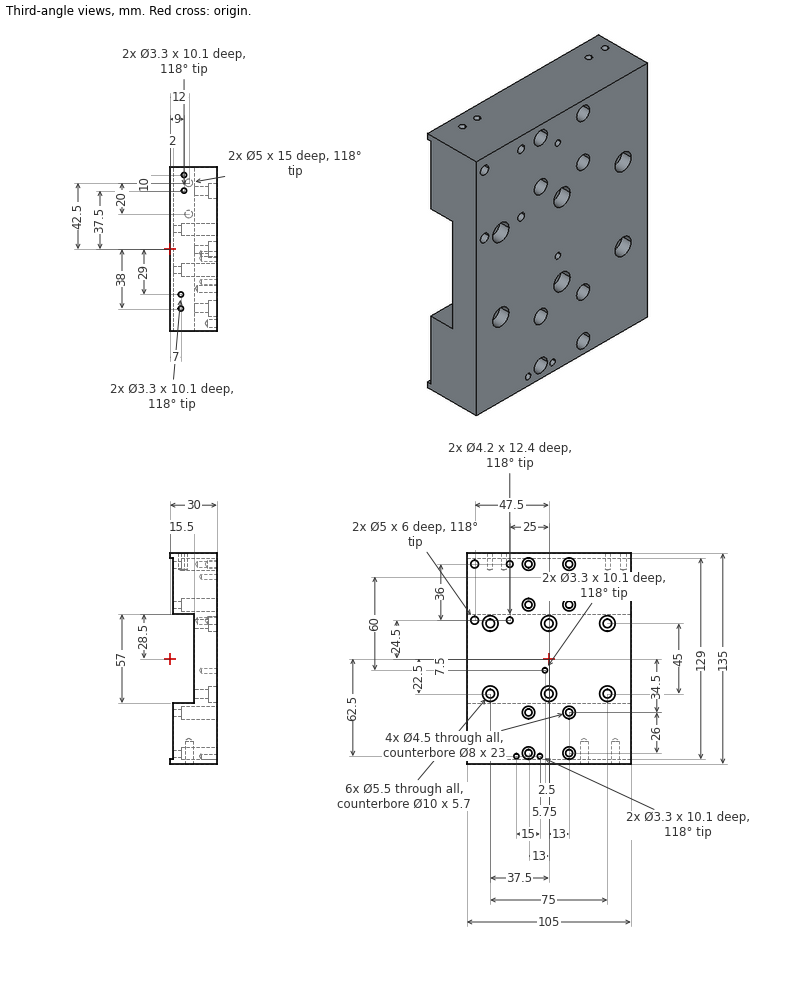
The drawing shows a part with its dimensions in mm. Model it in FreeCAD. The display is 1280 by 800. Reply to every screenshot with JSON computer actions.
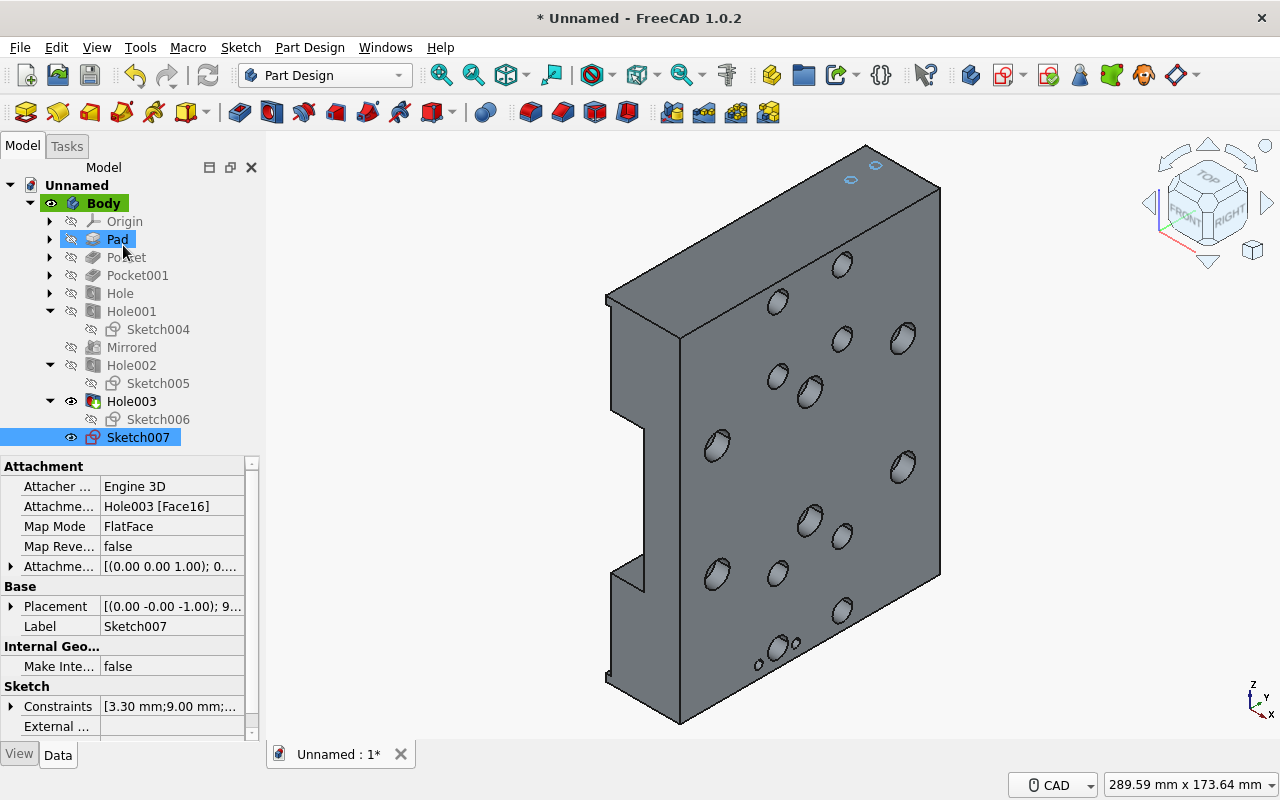
{"action": "left_click", "coordinate": [272, 112]}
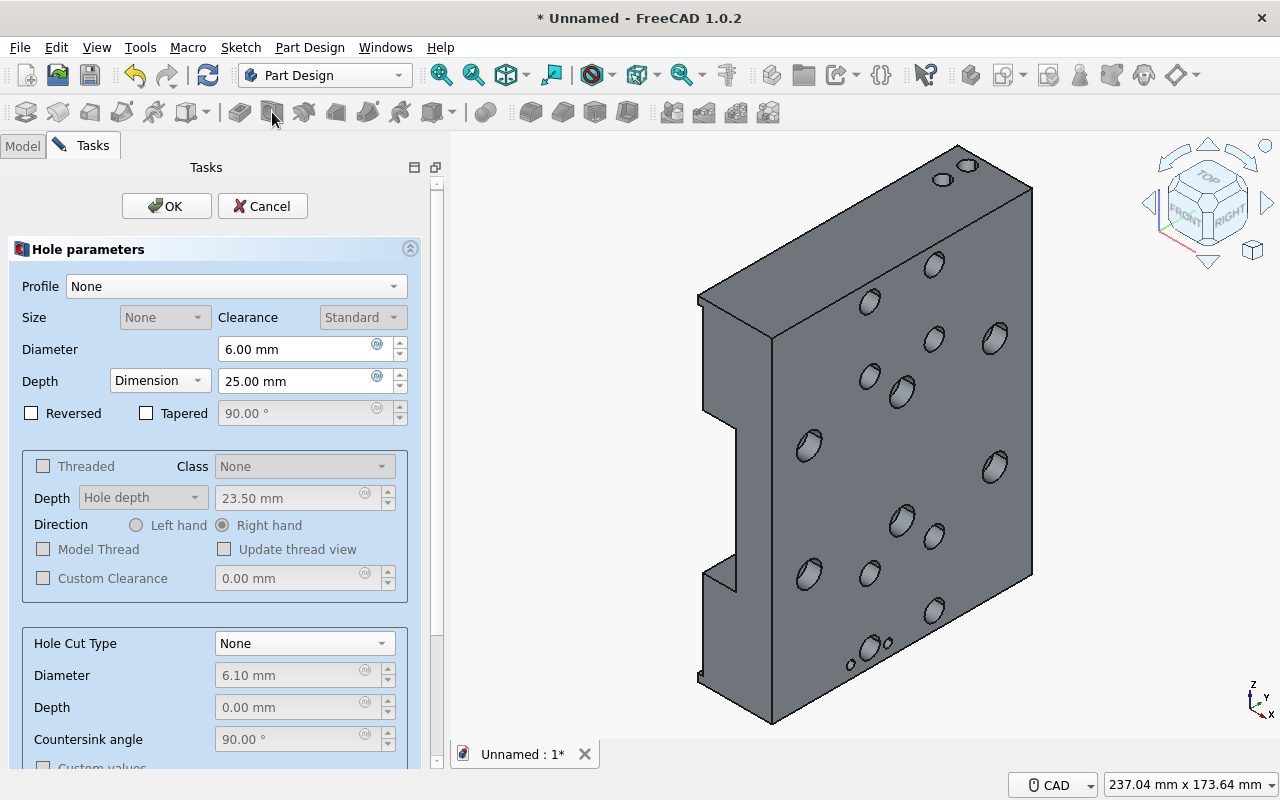
{"action": "triple_click", "coordinate": [305, 349]}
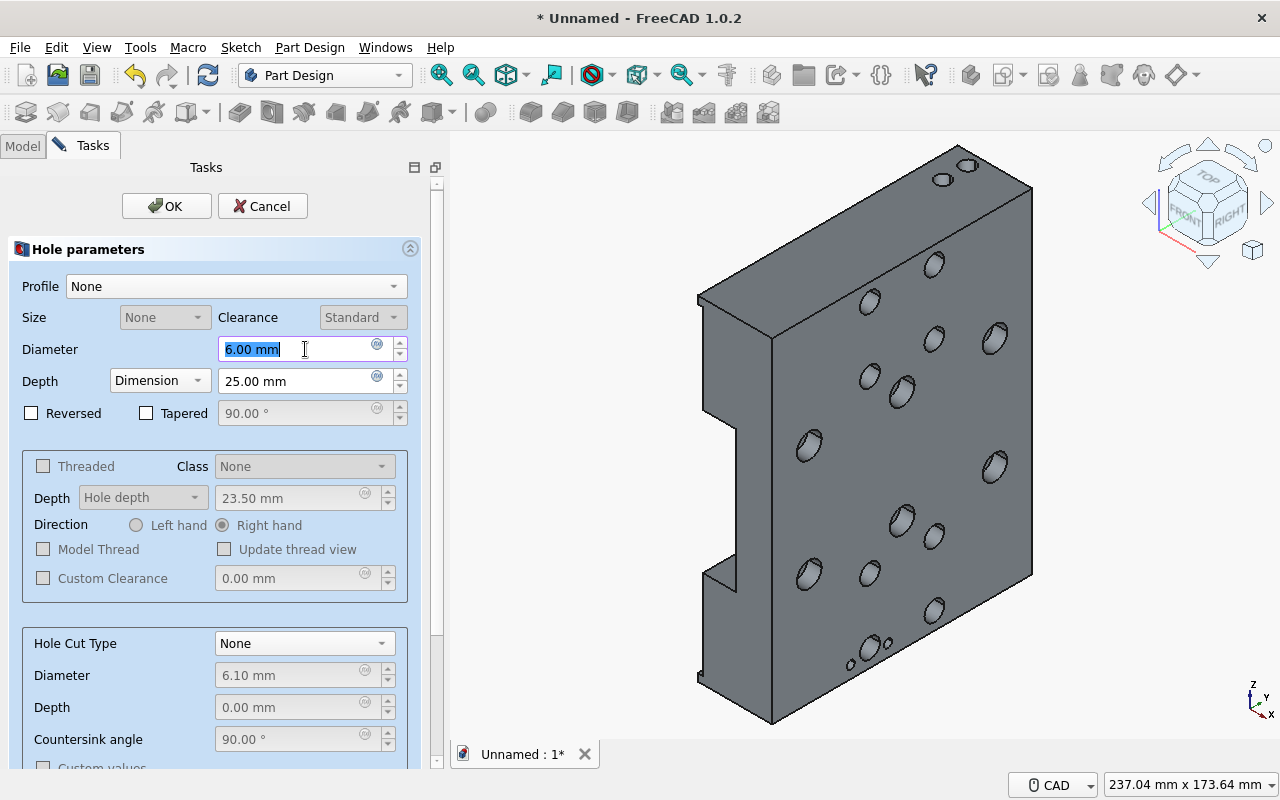
{"action": "type", "text": "3.3"}
{"action": "key", "text": "Tab"}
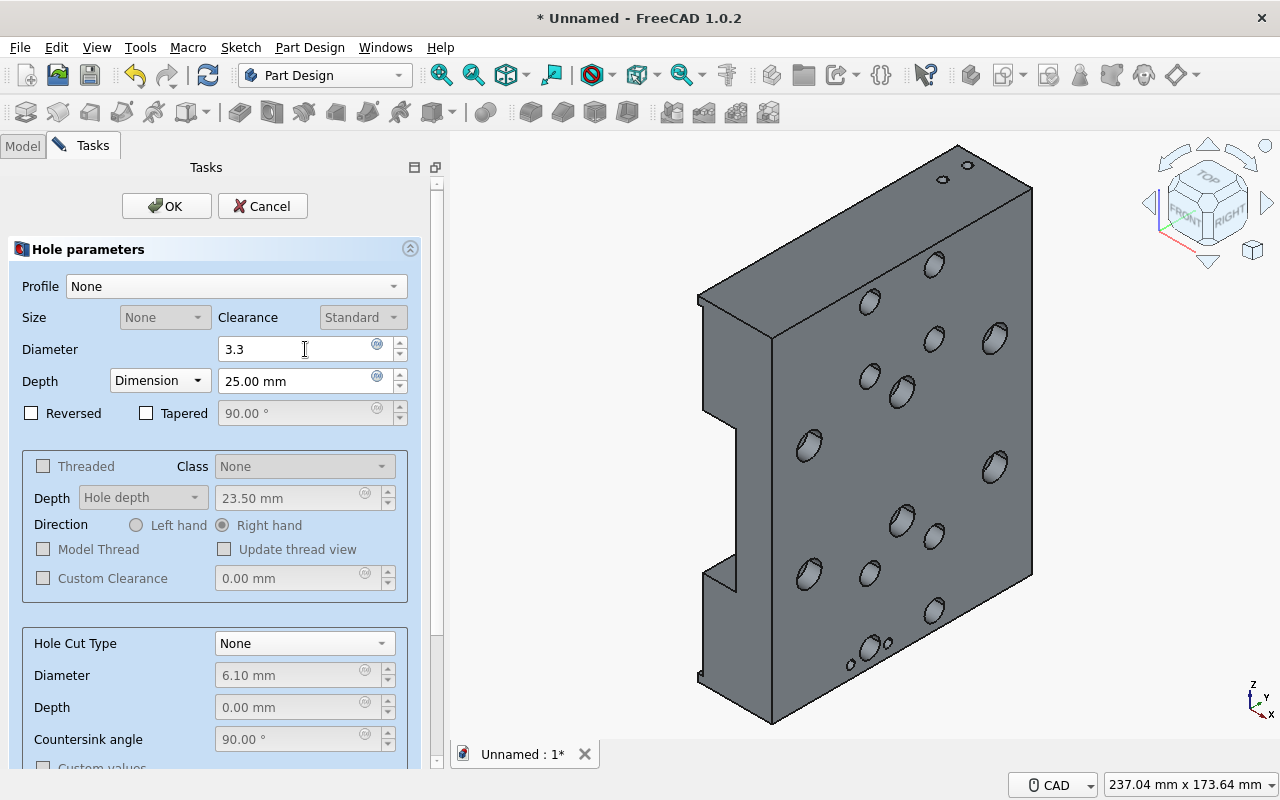
{"action": "triple_click", "coordinate": [305, 381]}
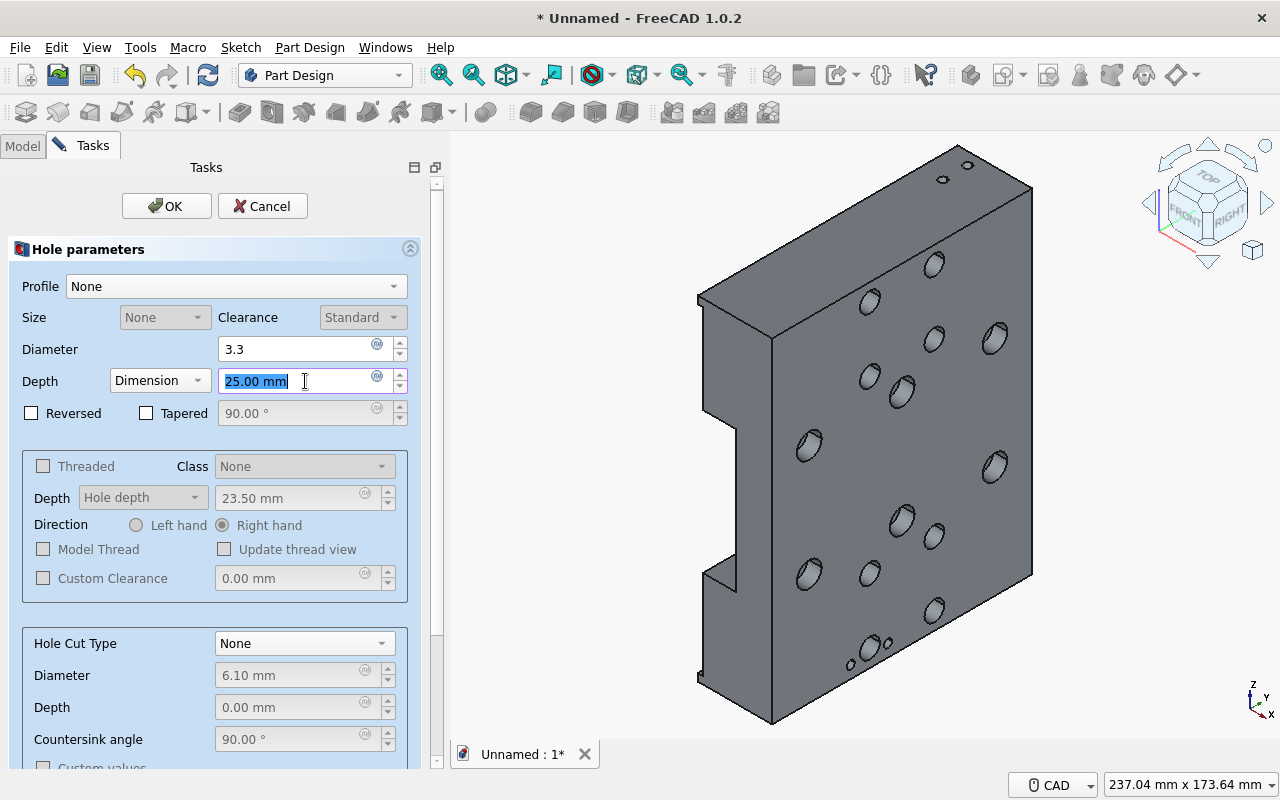
{"action": "type", "text": "10.1"}
{"action": "key", "text": "Tab"}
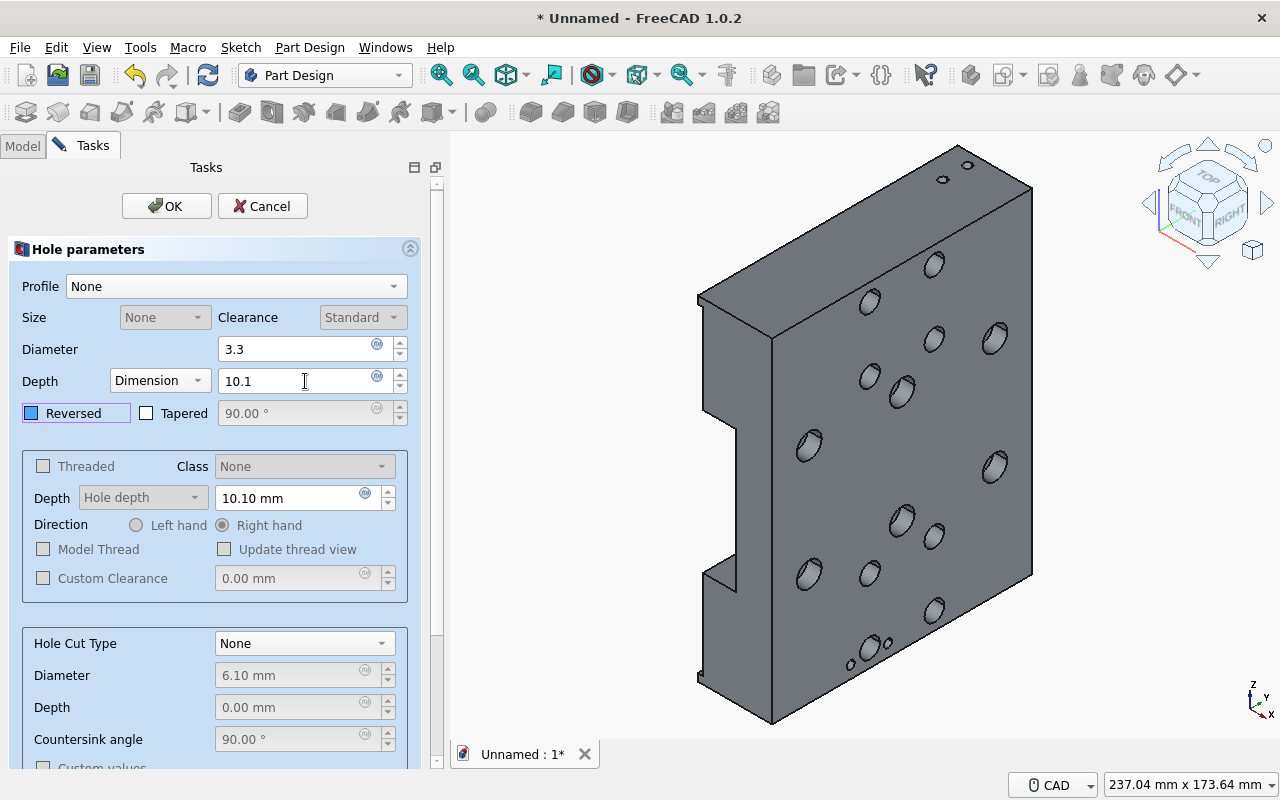
{"action": "left_click", "coordinate": [167, 206]}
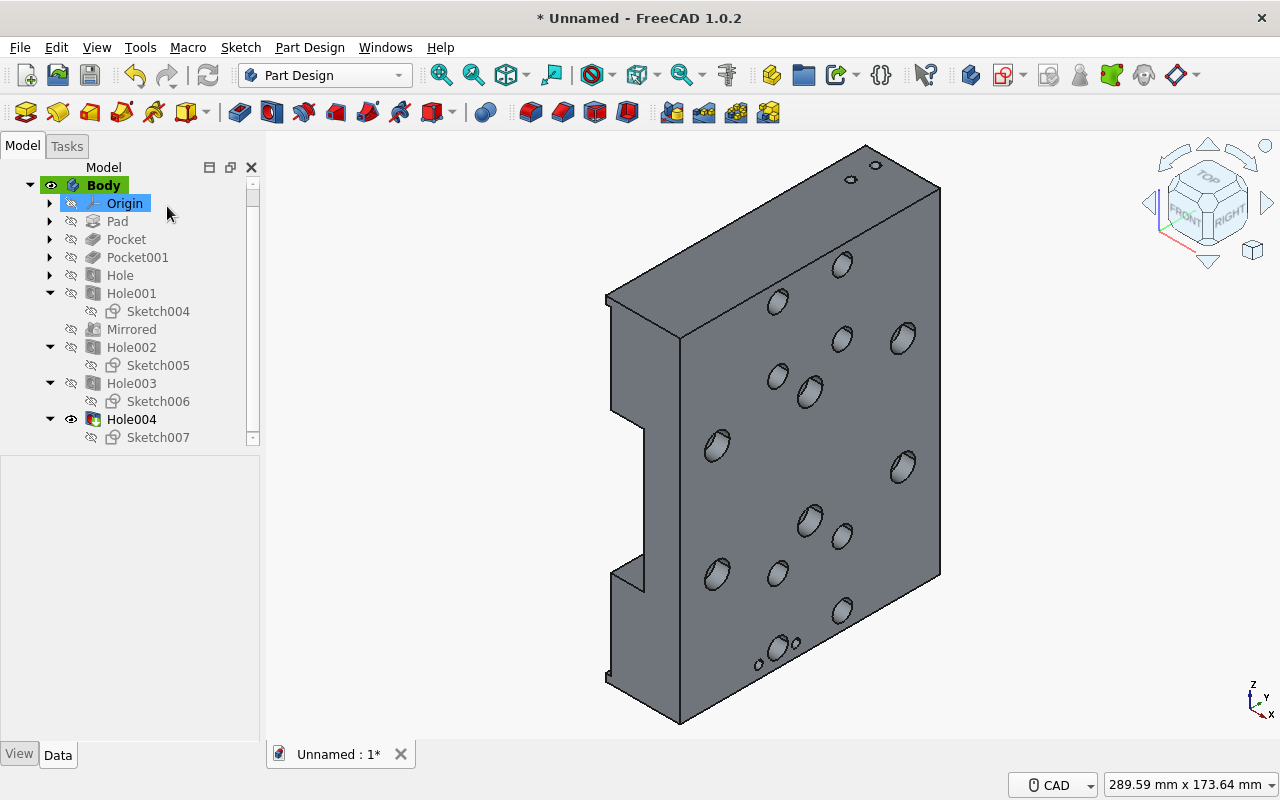
{"action": "left_click", "coordinate": [810, 220]}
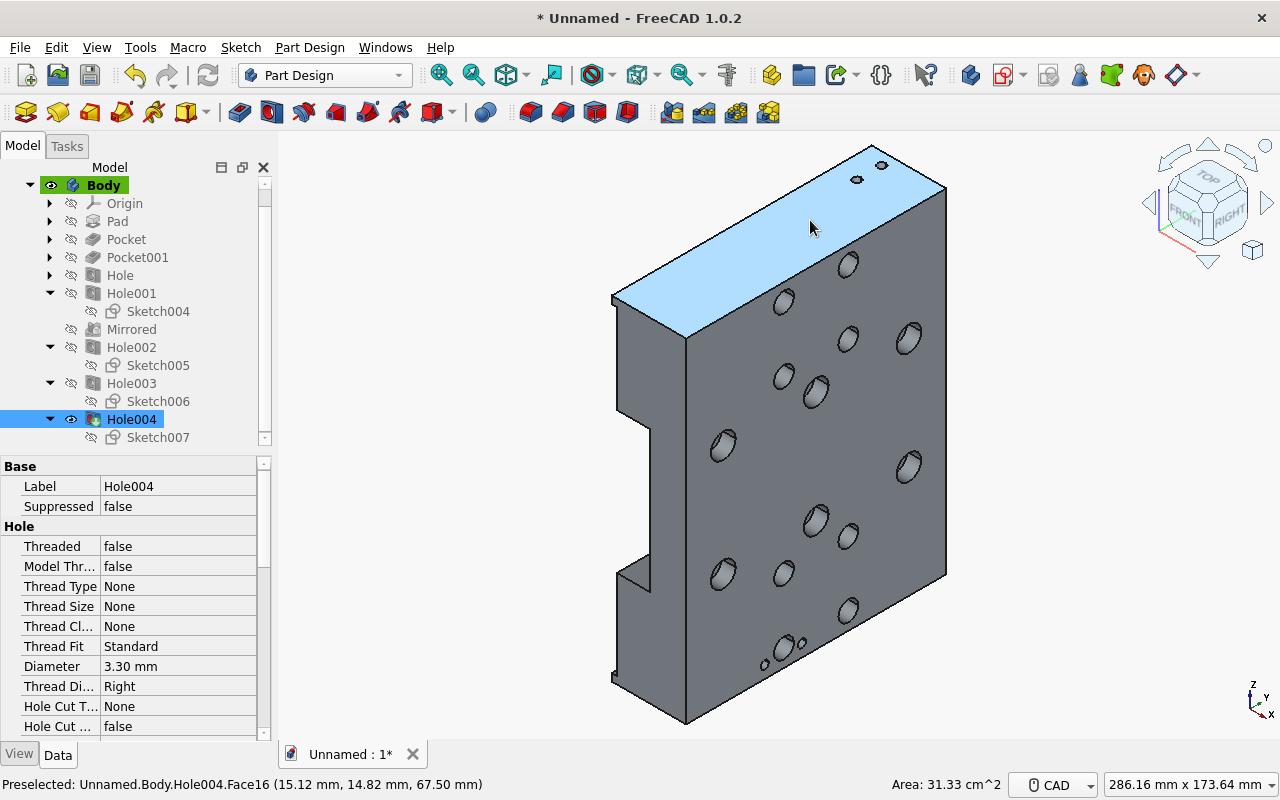
{"action": "left_click", "coordinate": [1004, 76]}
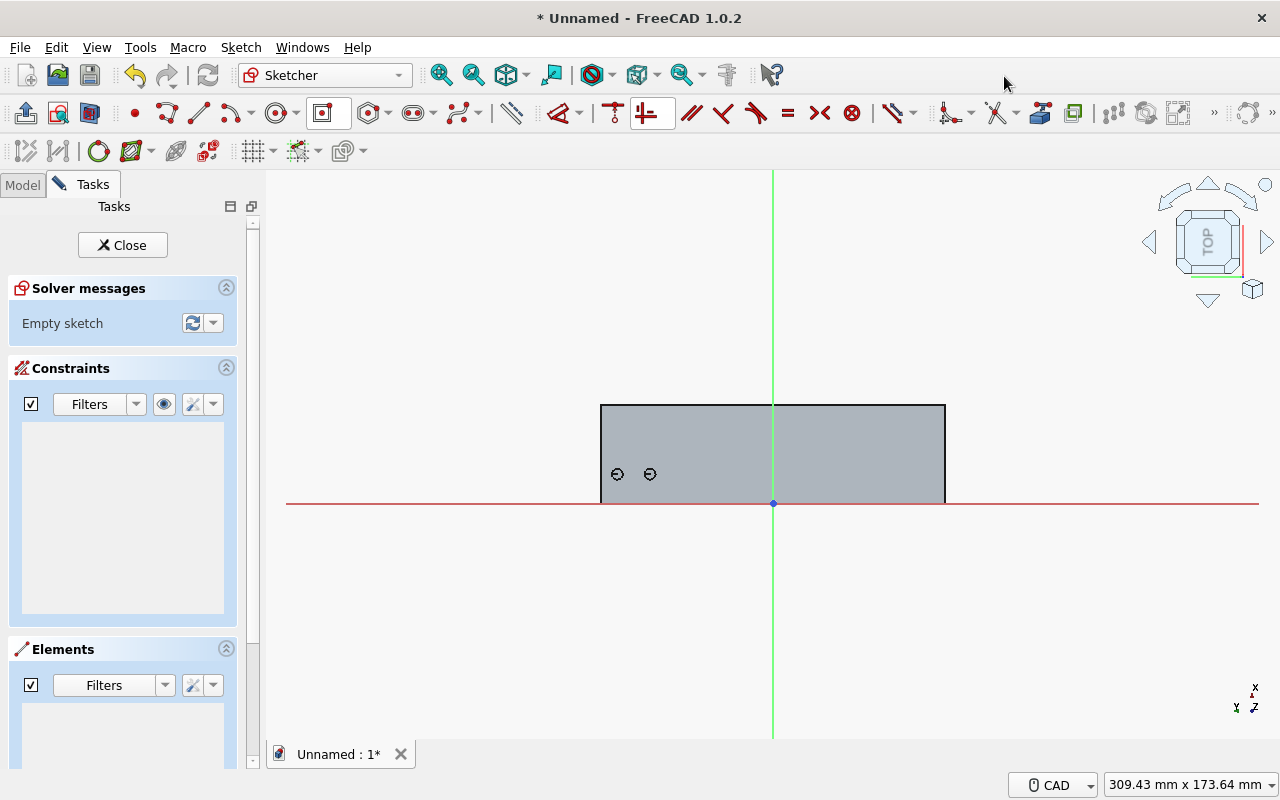
{"action": "scroll", "coordinate": [897, 483], "scroll_direction": "up", "scroll_amount": 13}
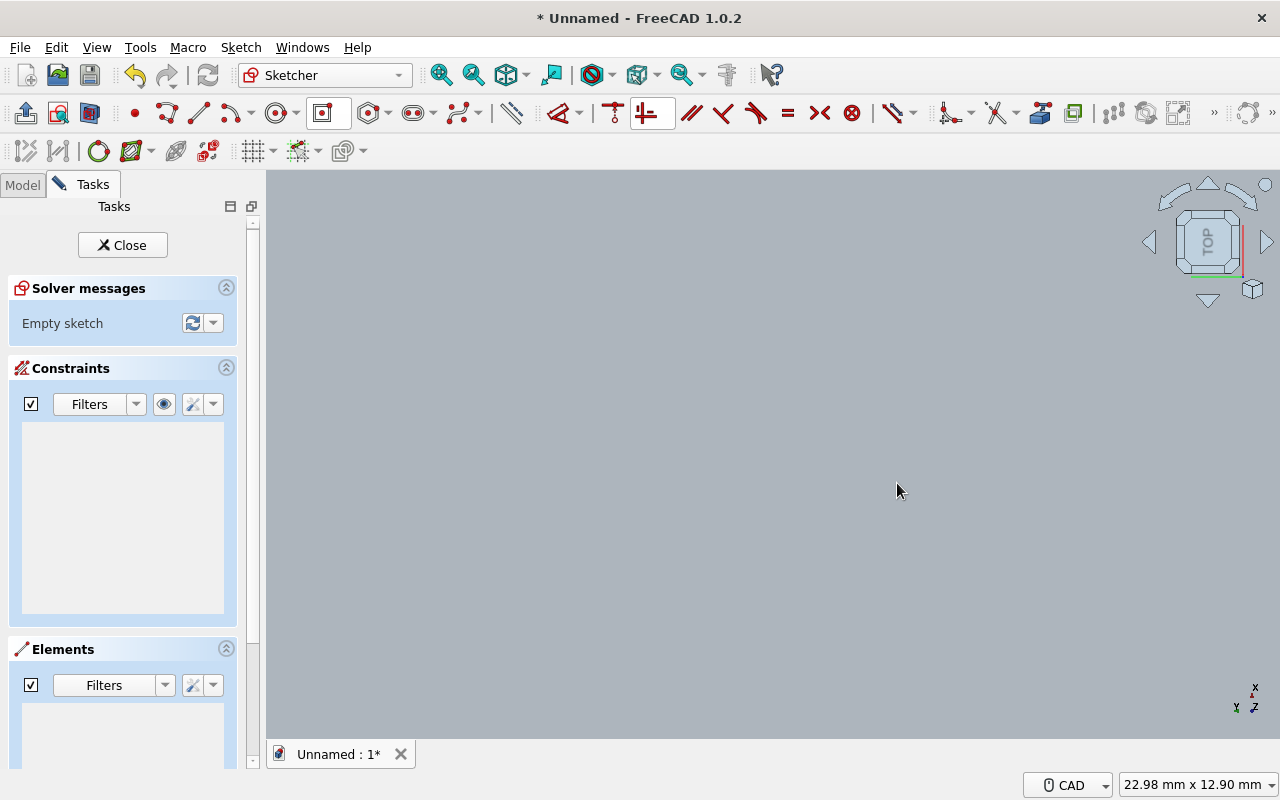
{"action": "left_click", "coordinate": [276, 114]}